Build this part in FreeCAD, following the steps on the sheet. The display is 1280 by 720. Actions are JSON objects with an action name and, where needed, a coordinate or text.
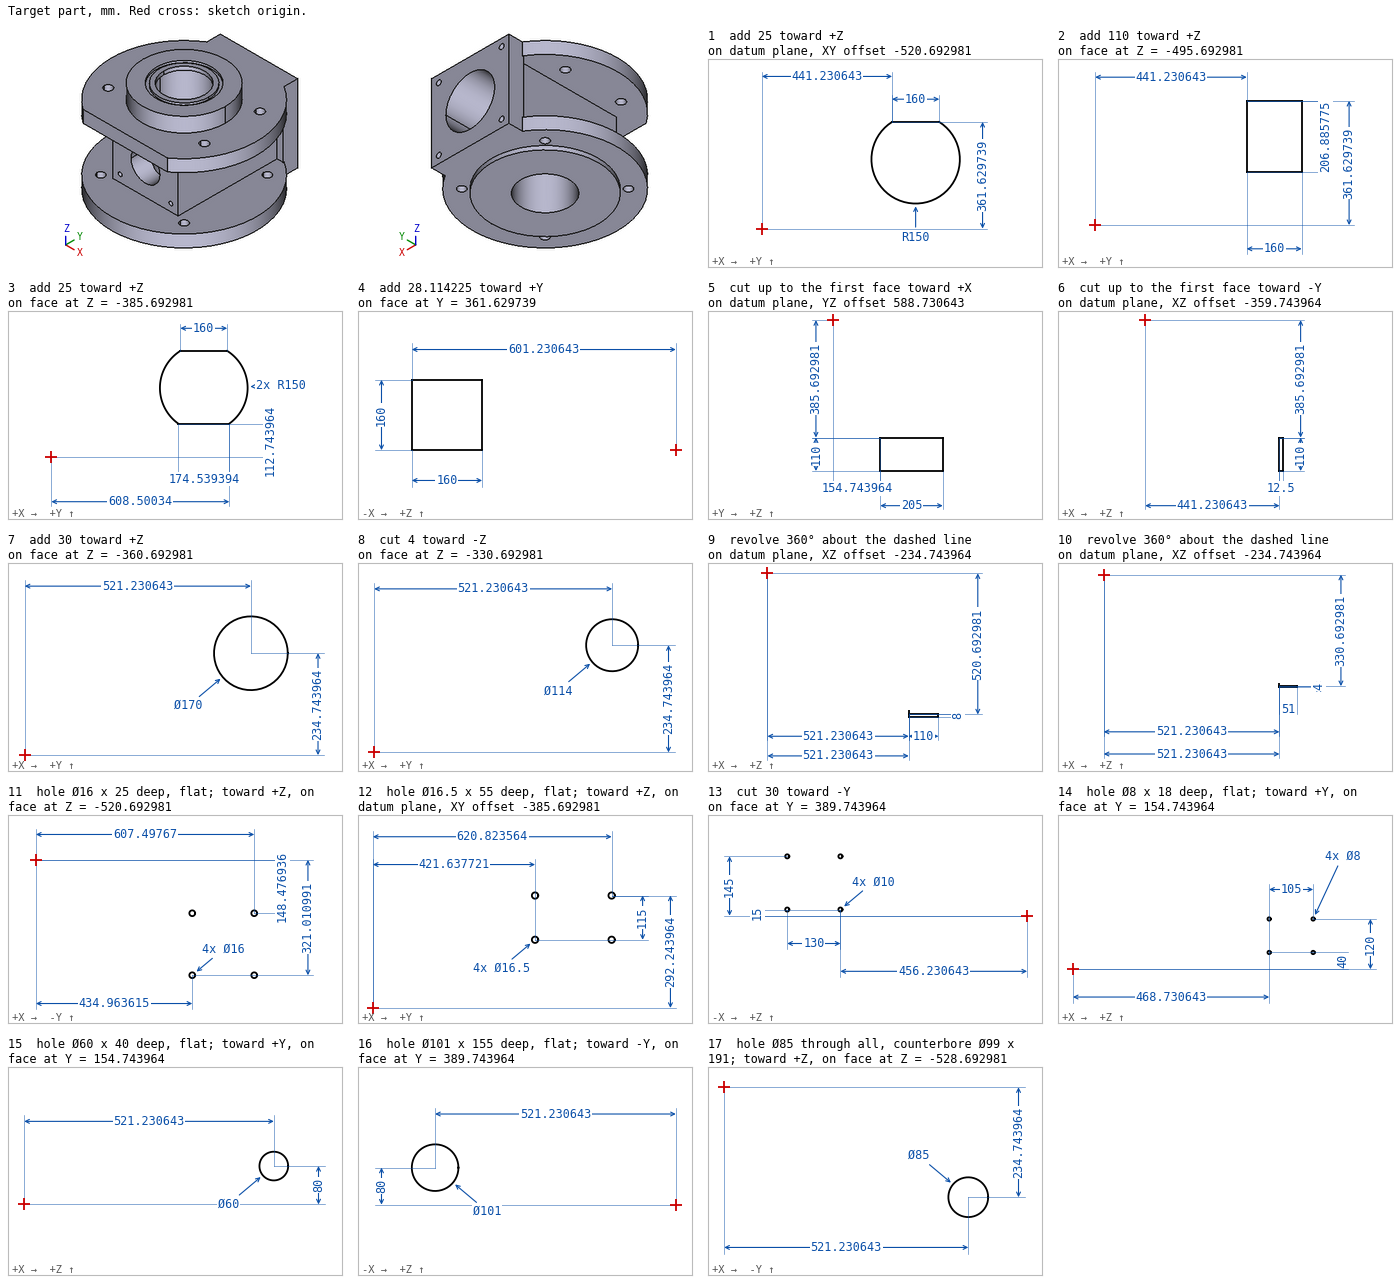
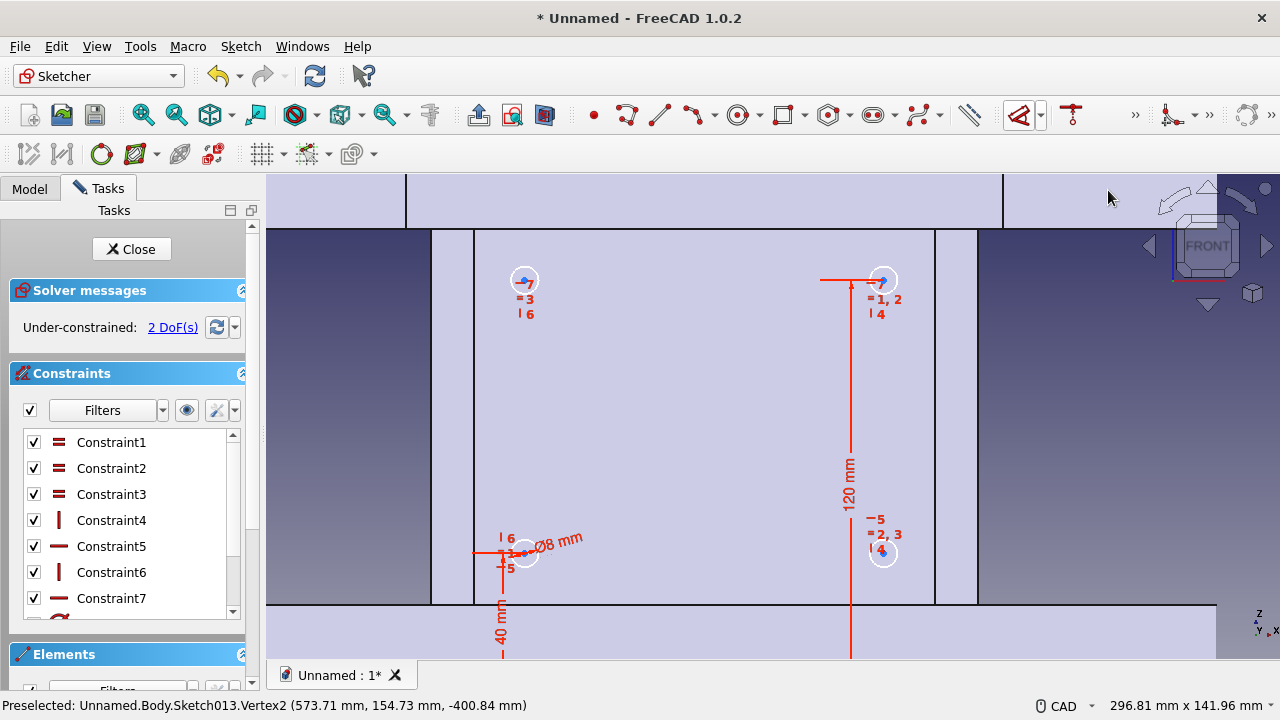
{"action": "left_click", "coordinate": [525, 553]}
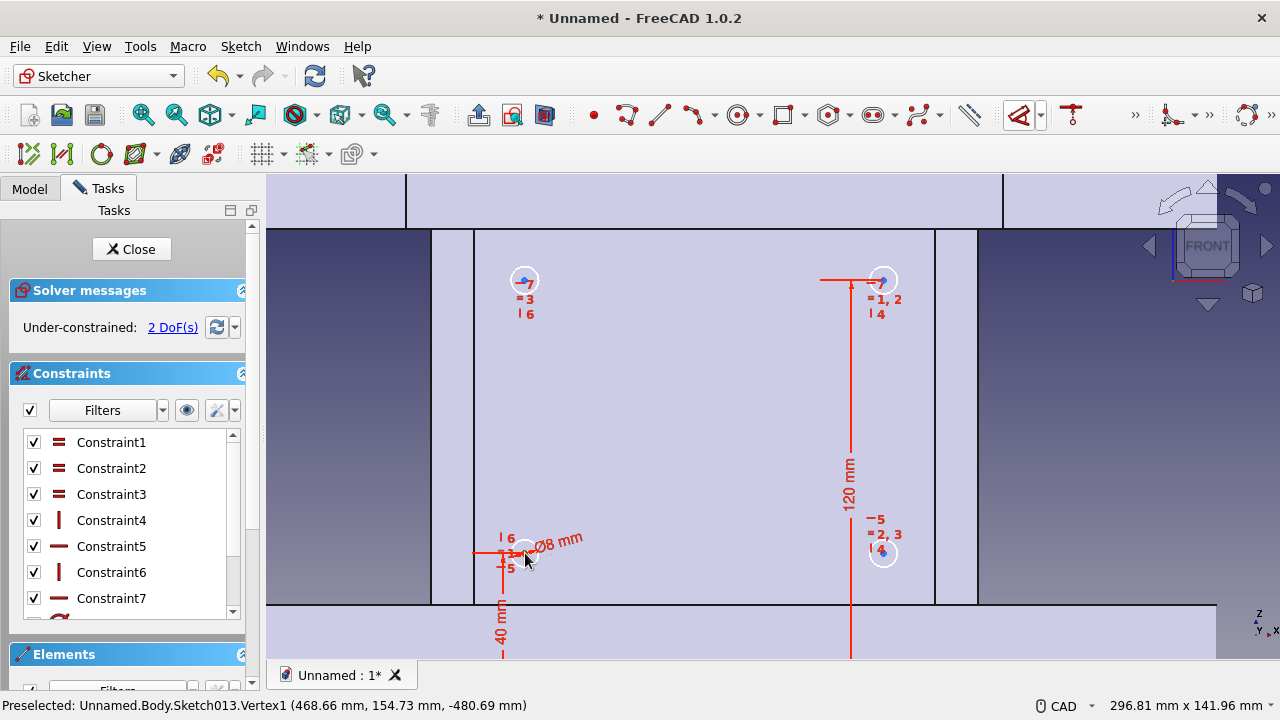
{"action": "left_click", "coordinate": [884, 280]}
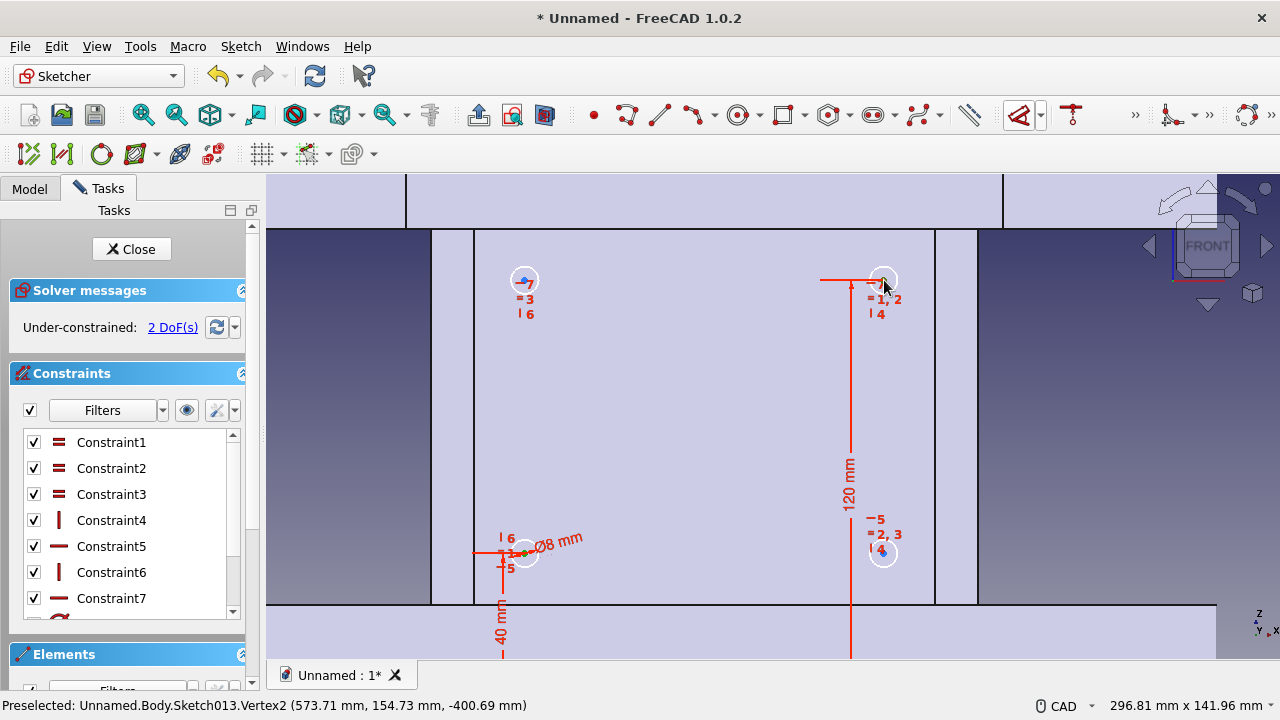
{"action": "left_click", "coordinate": [1040, 116]}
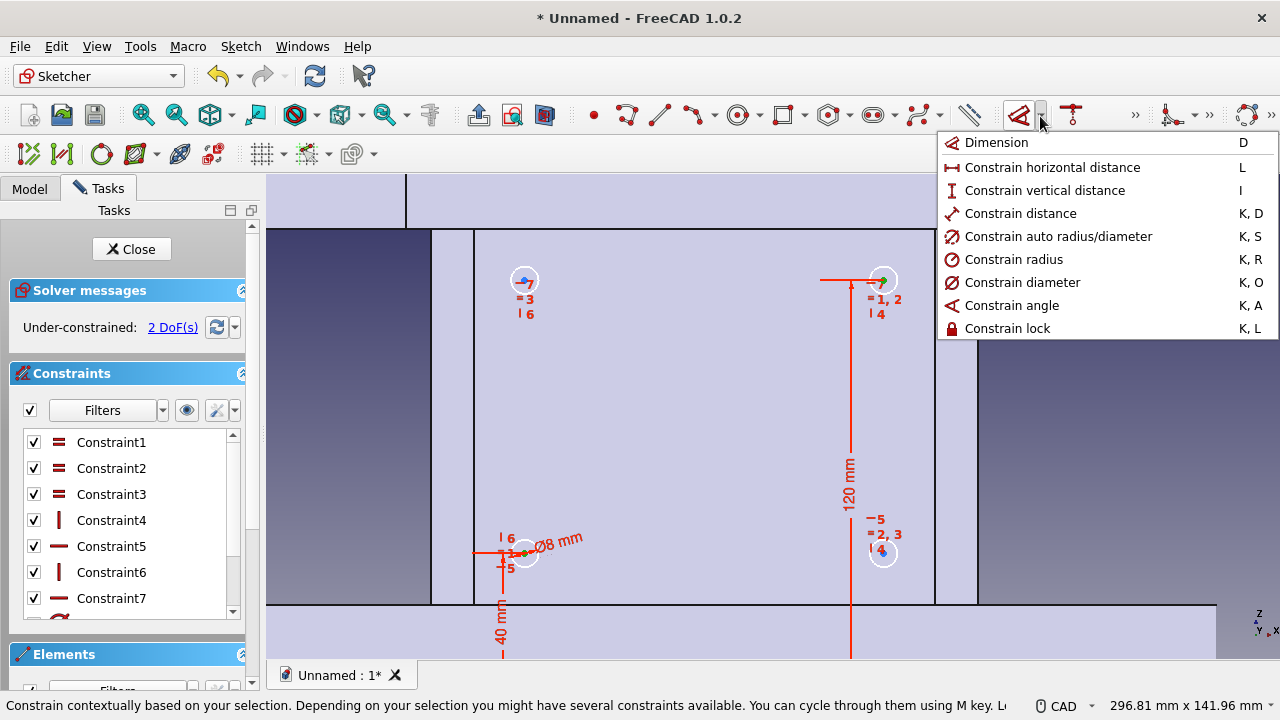
{"action": "left_click", "coordinate": [1108, 168]}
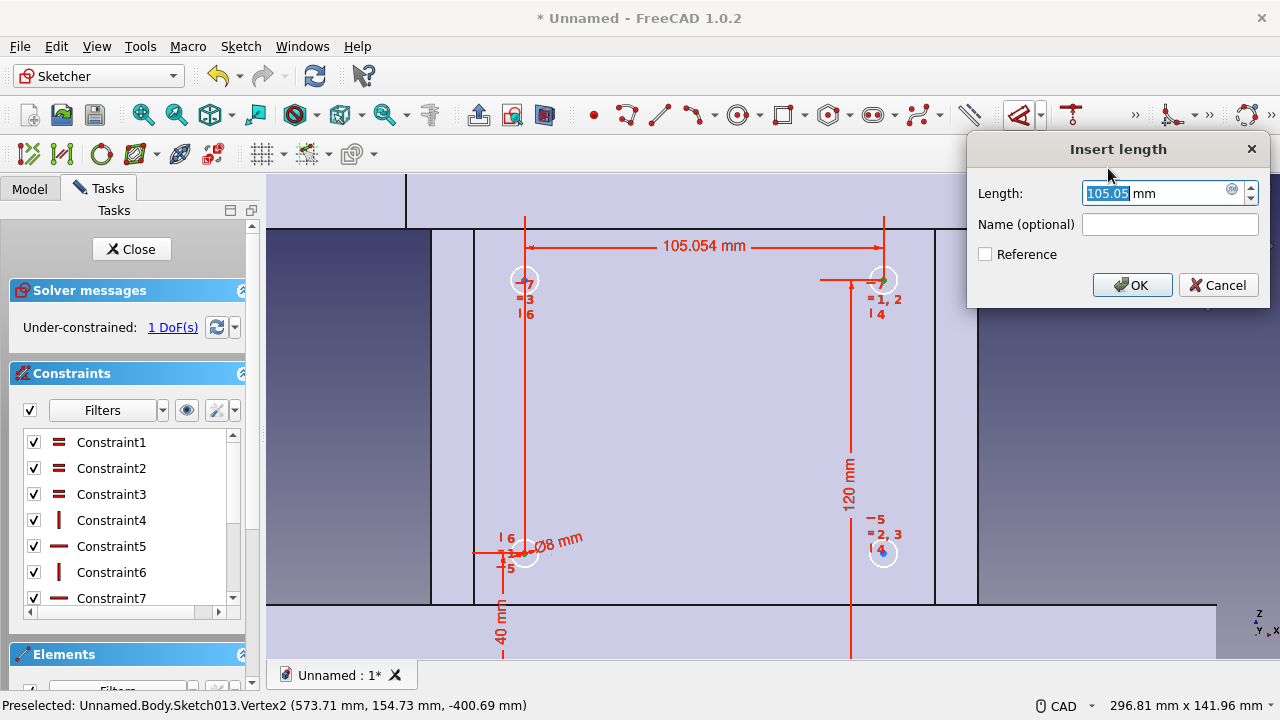
{"action": "type", "text": "105"}
{"action": "key", "text": "Return"}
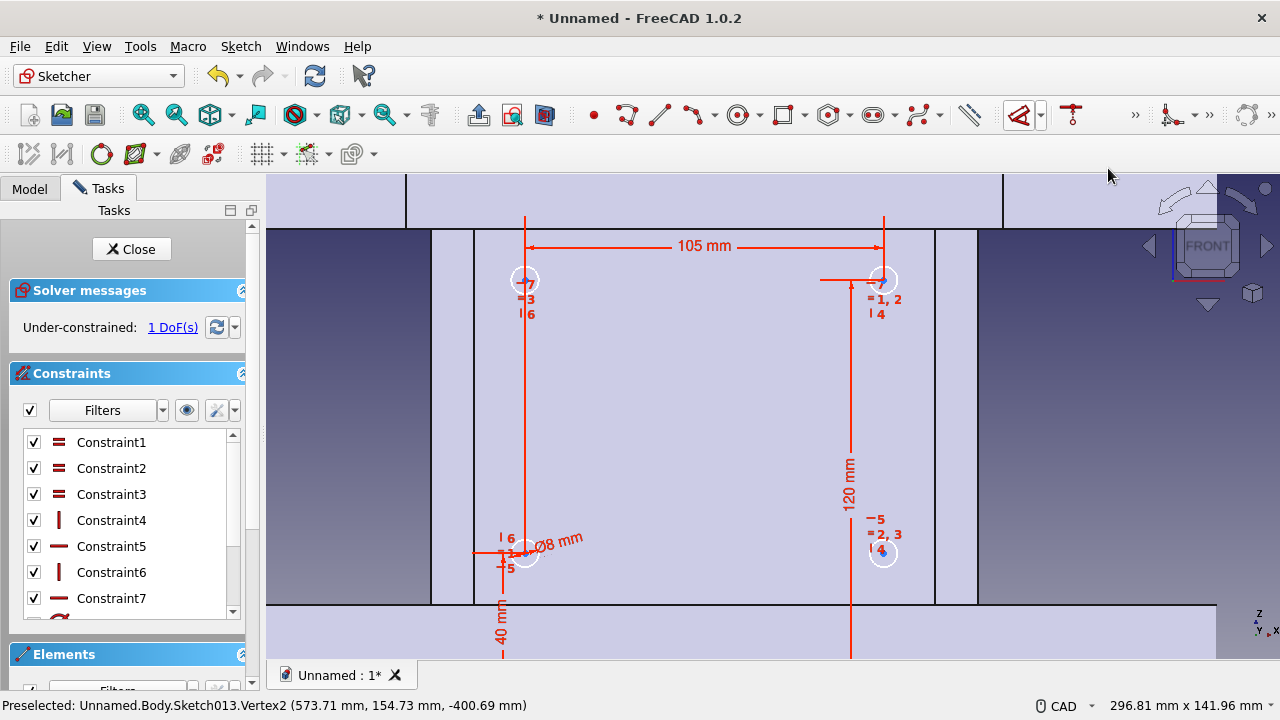
{"action": "left_click", "coordinate": [525, 553]}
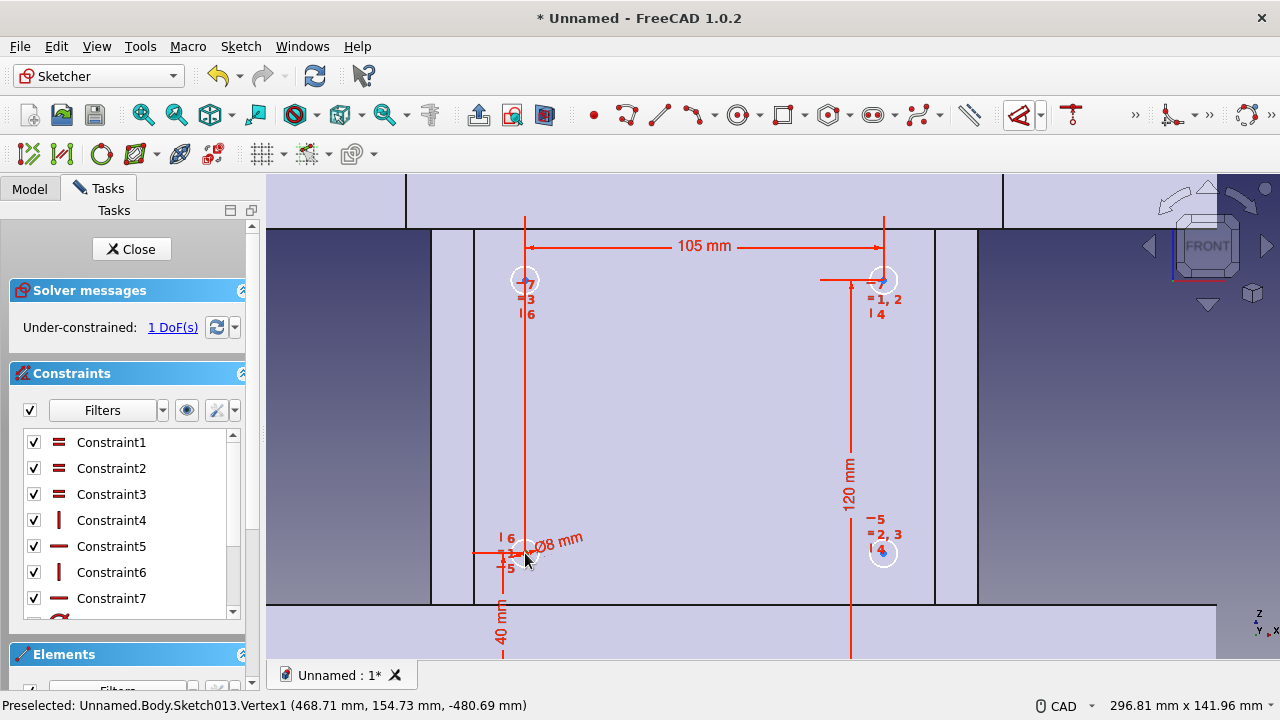
{"action": "left_click", "coordinate": [1040, 116]}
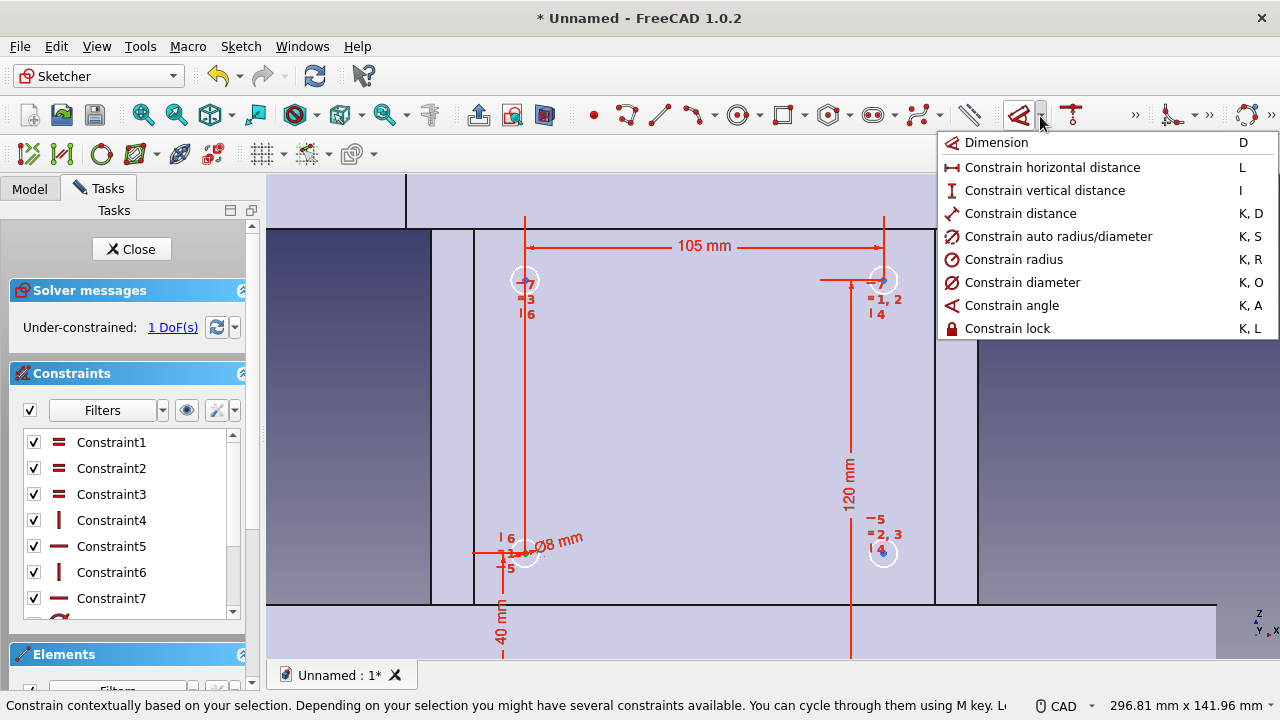
{"action": "left_click", "coordinate": [1108, 168]}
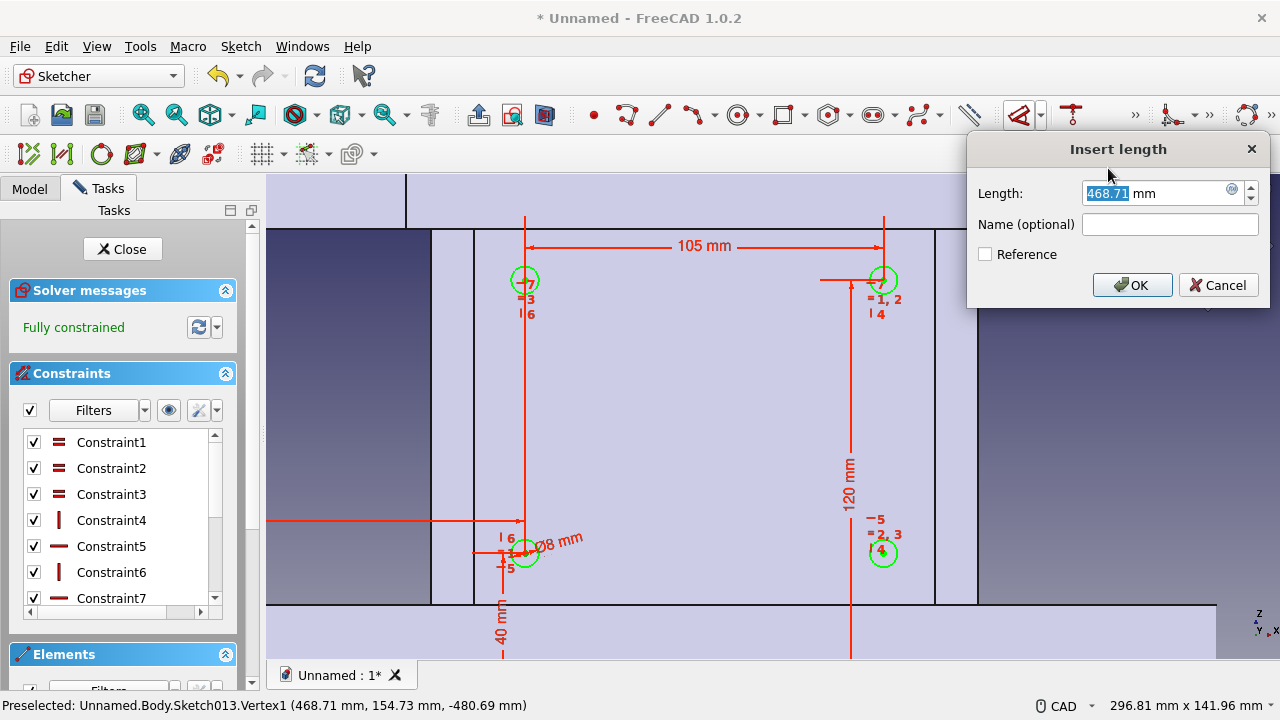
{"action": "type", "text": "468.730643"}
{"action": "key", "text": "Return"}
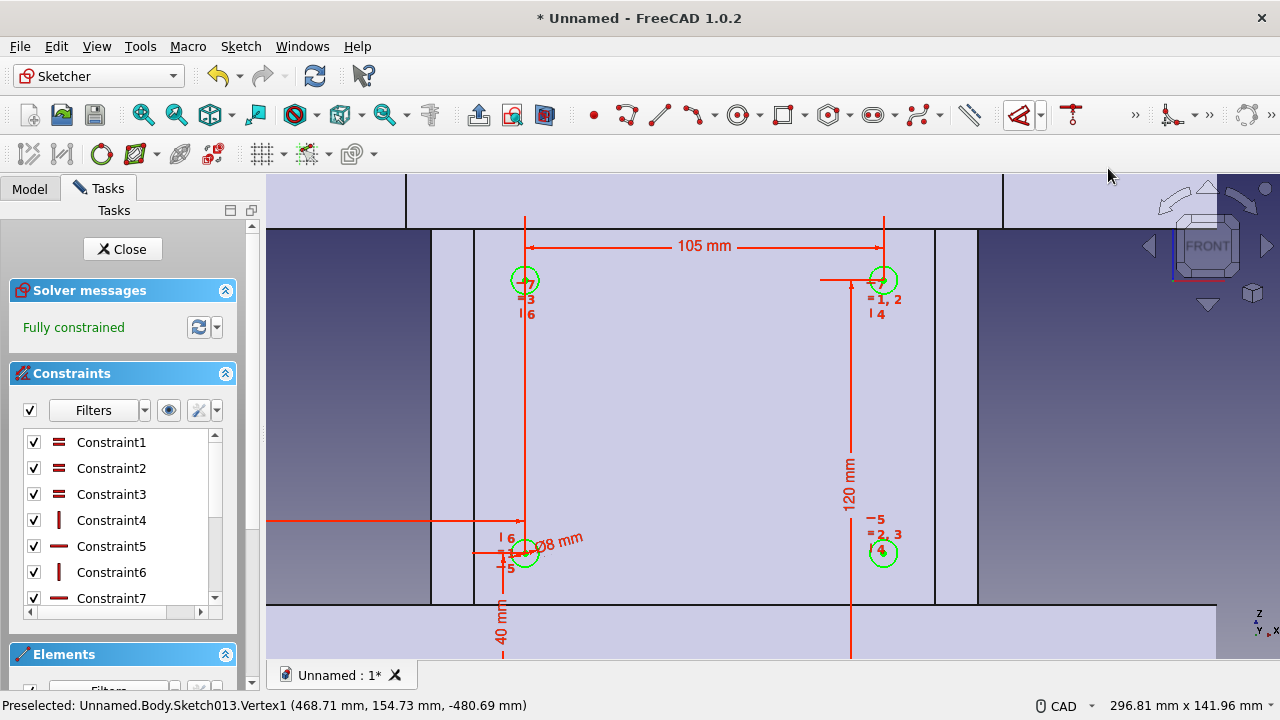
{"action": "left_click", "coordinate": [123, 249]}